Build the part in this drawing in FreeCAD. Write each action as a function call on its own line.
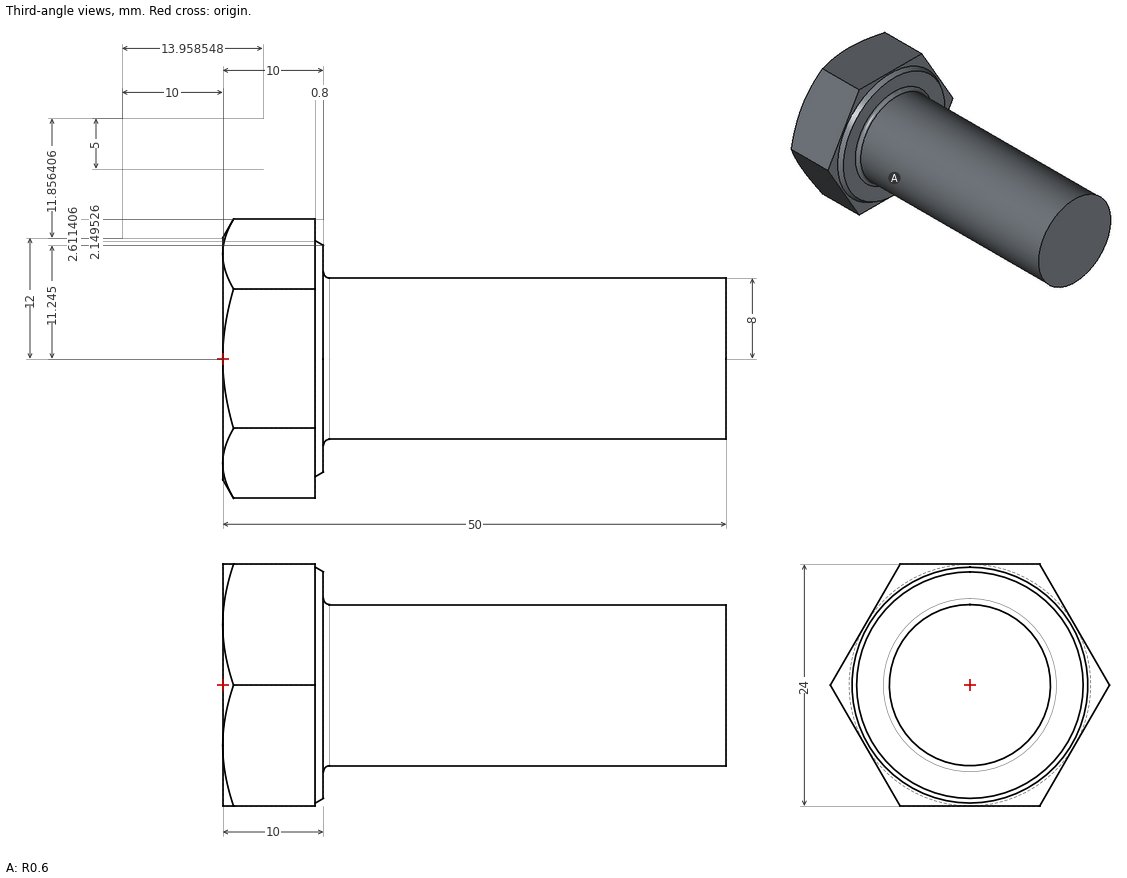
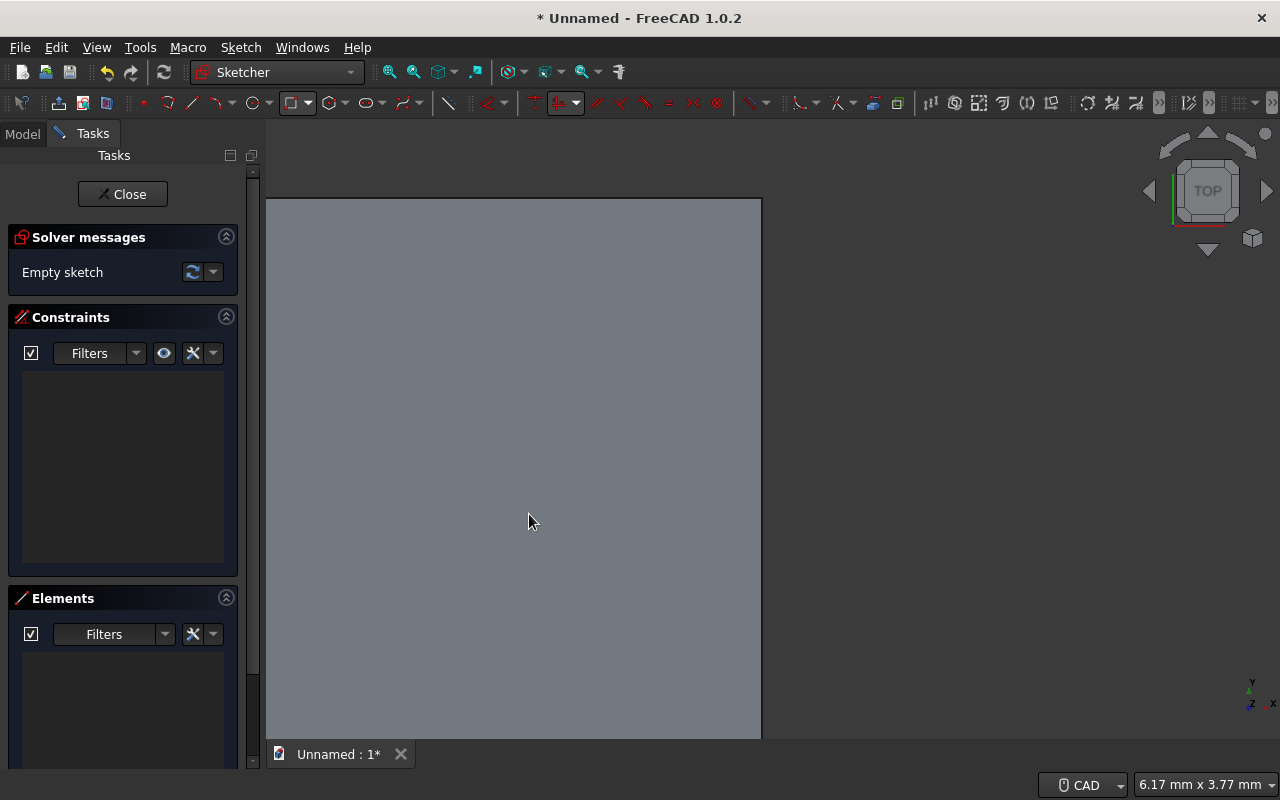
click(168, 104)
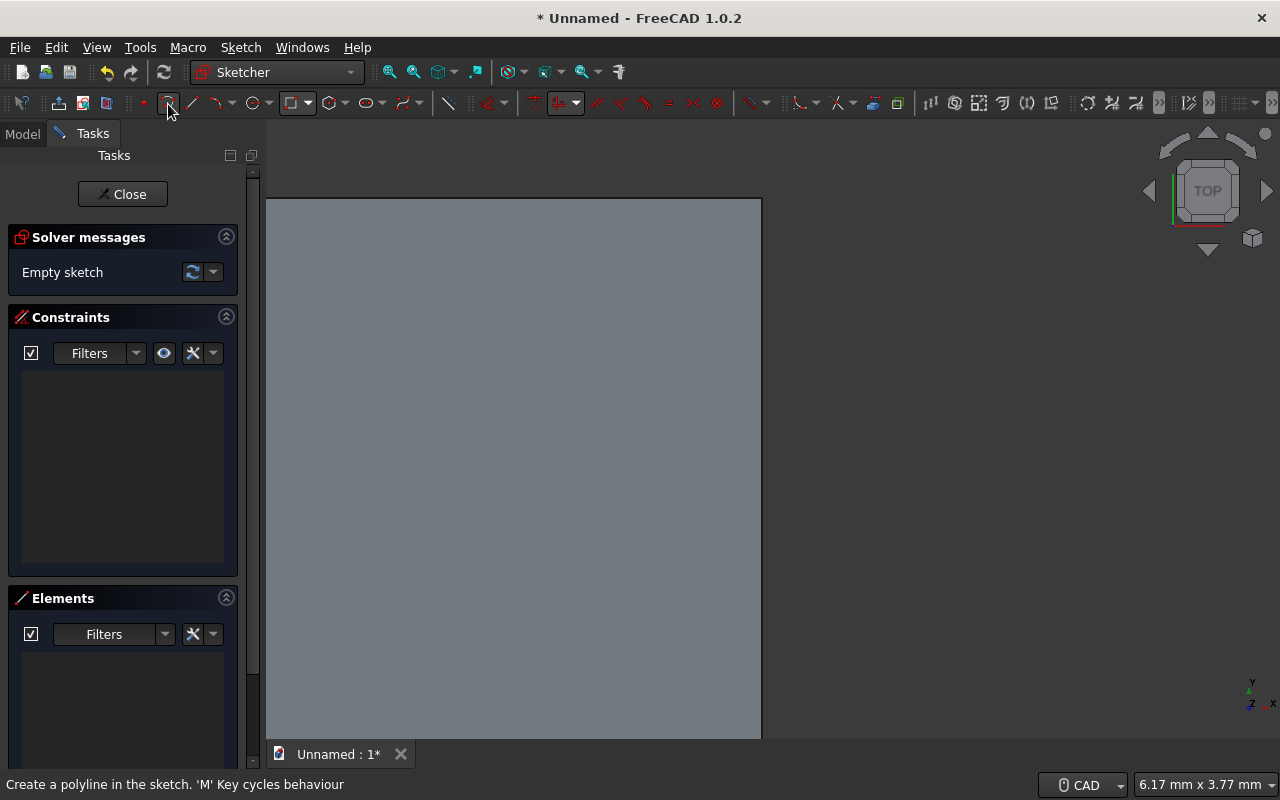
click(630, 552)
click(762, 628)
click(762, 198)
click(630, 198)
click(630, 553)
key(Escape)
key(Escape)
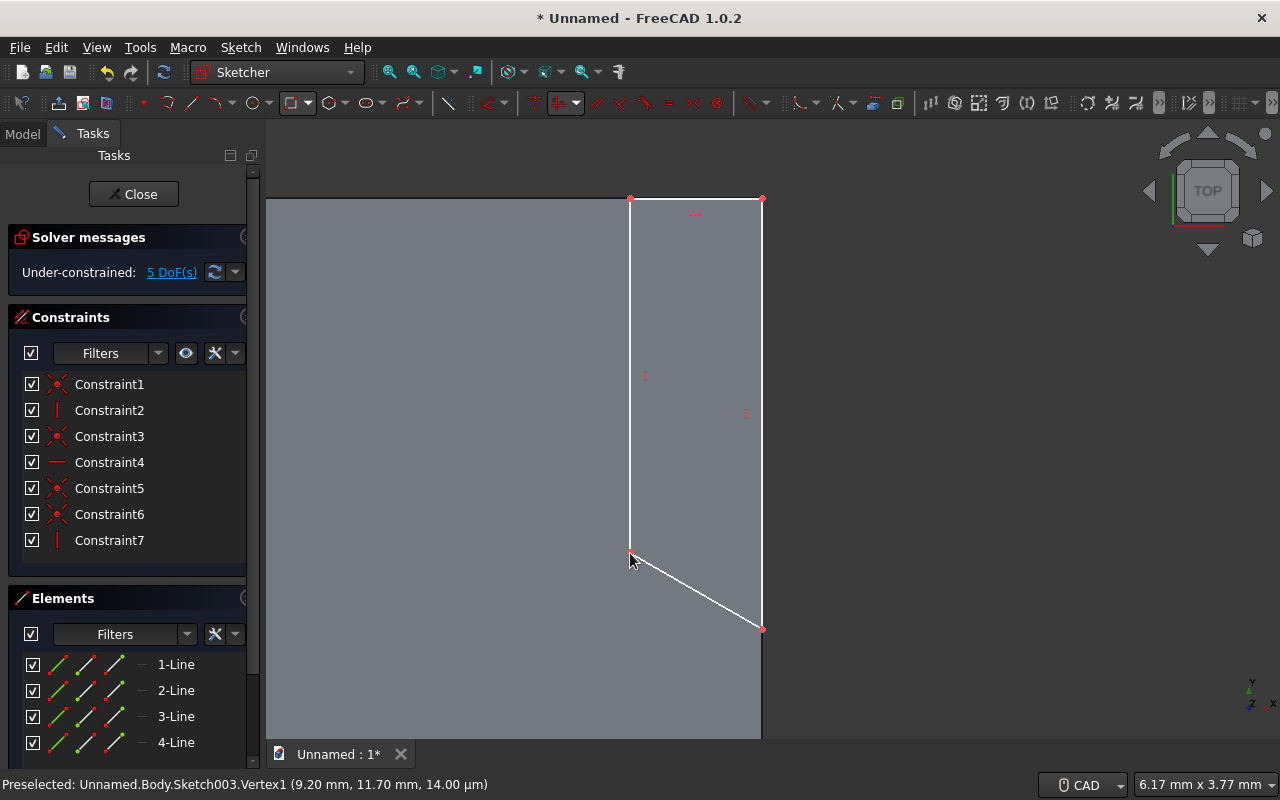
click(488, 104)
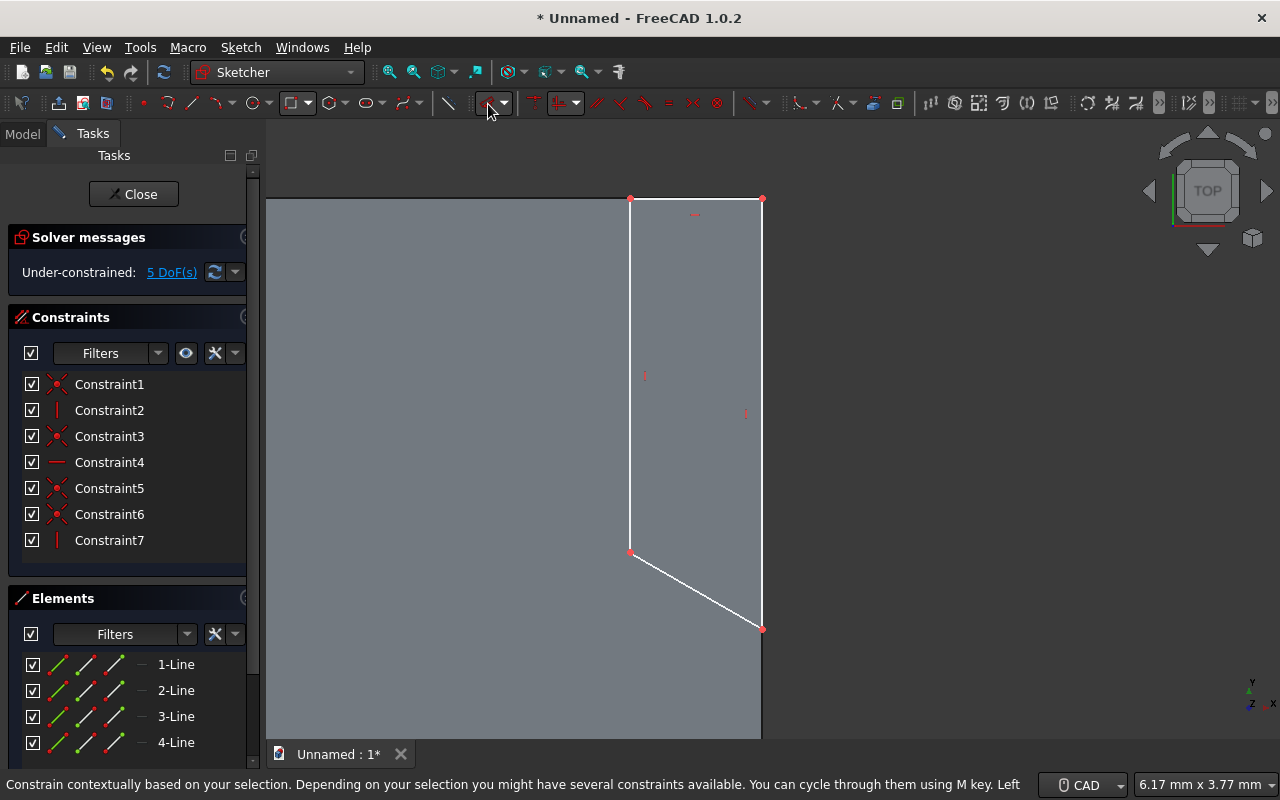
click(722, 199)
click(696, 165)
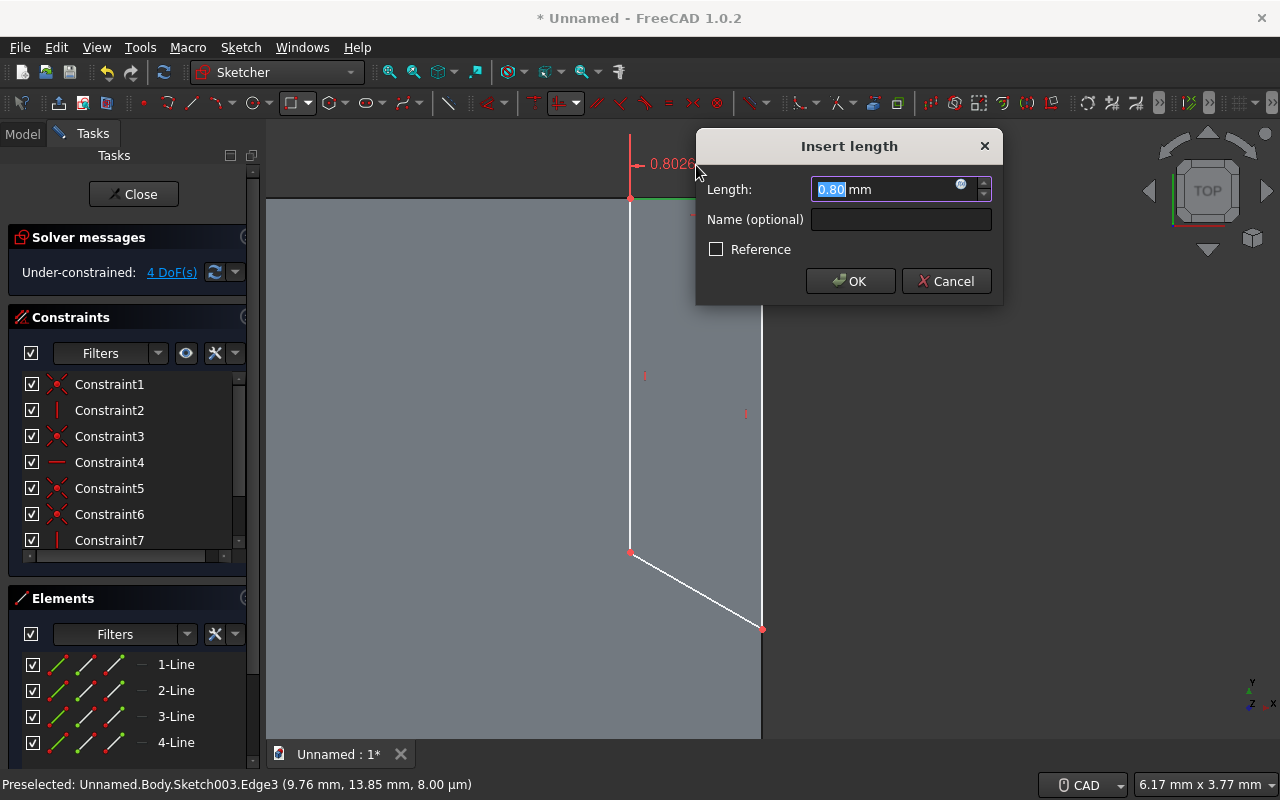
text(0.8)
key(Return)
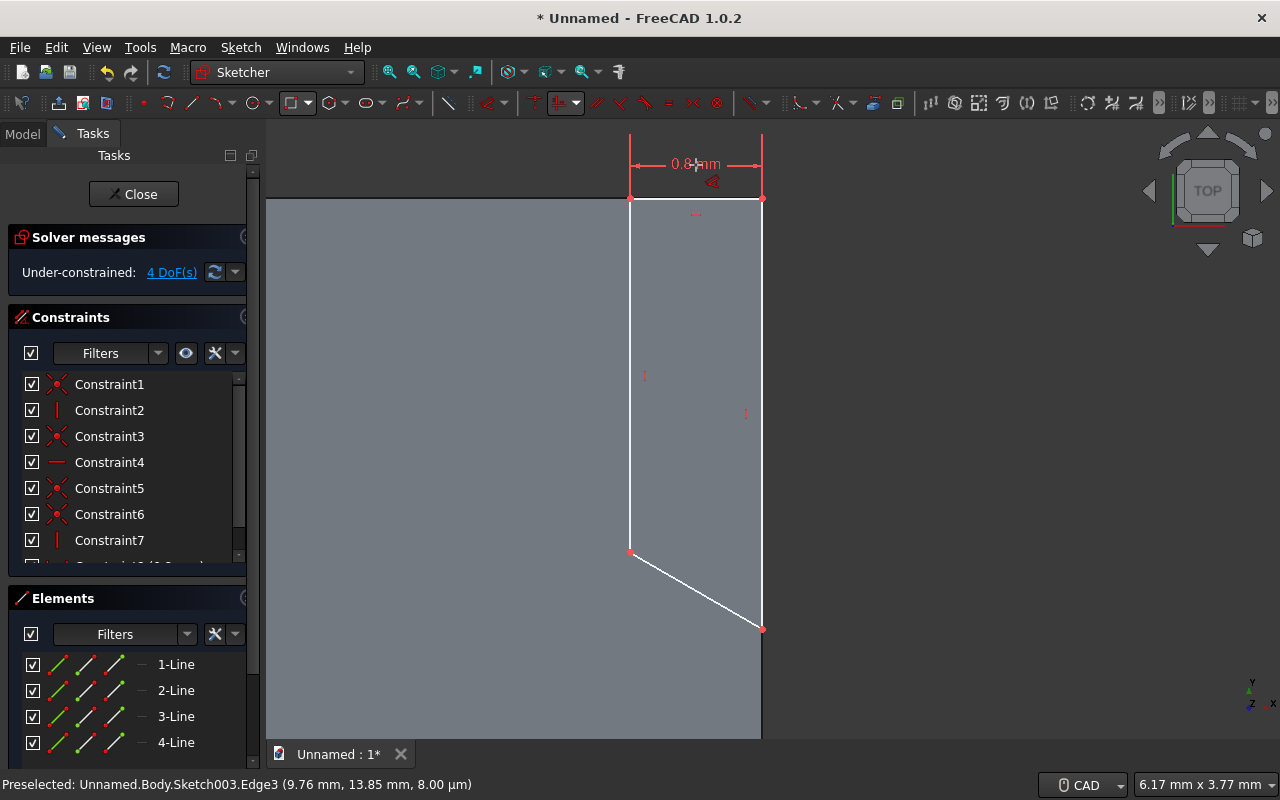
click(762, 629)
click(528, 595)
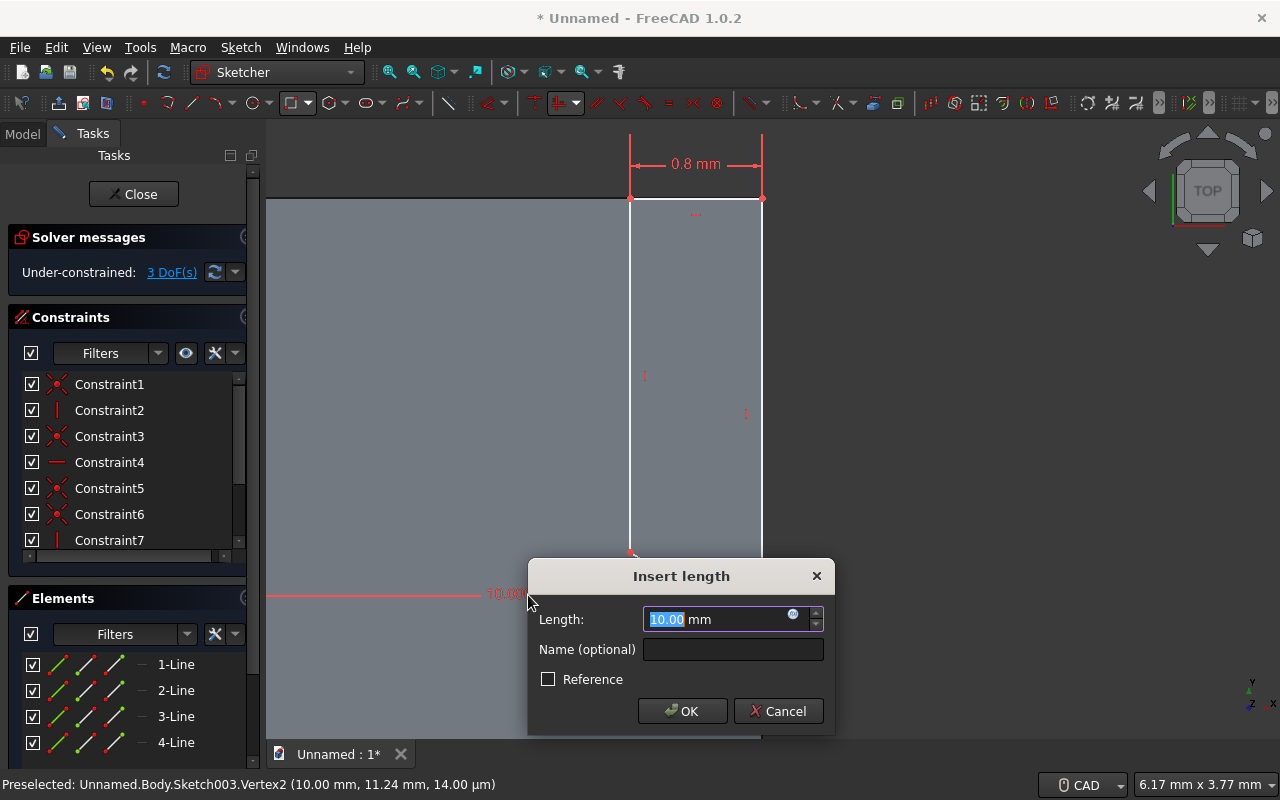
text(10)
key(Return)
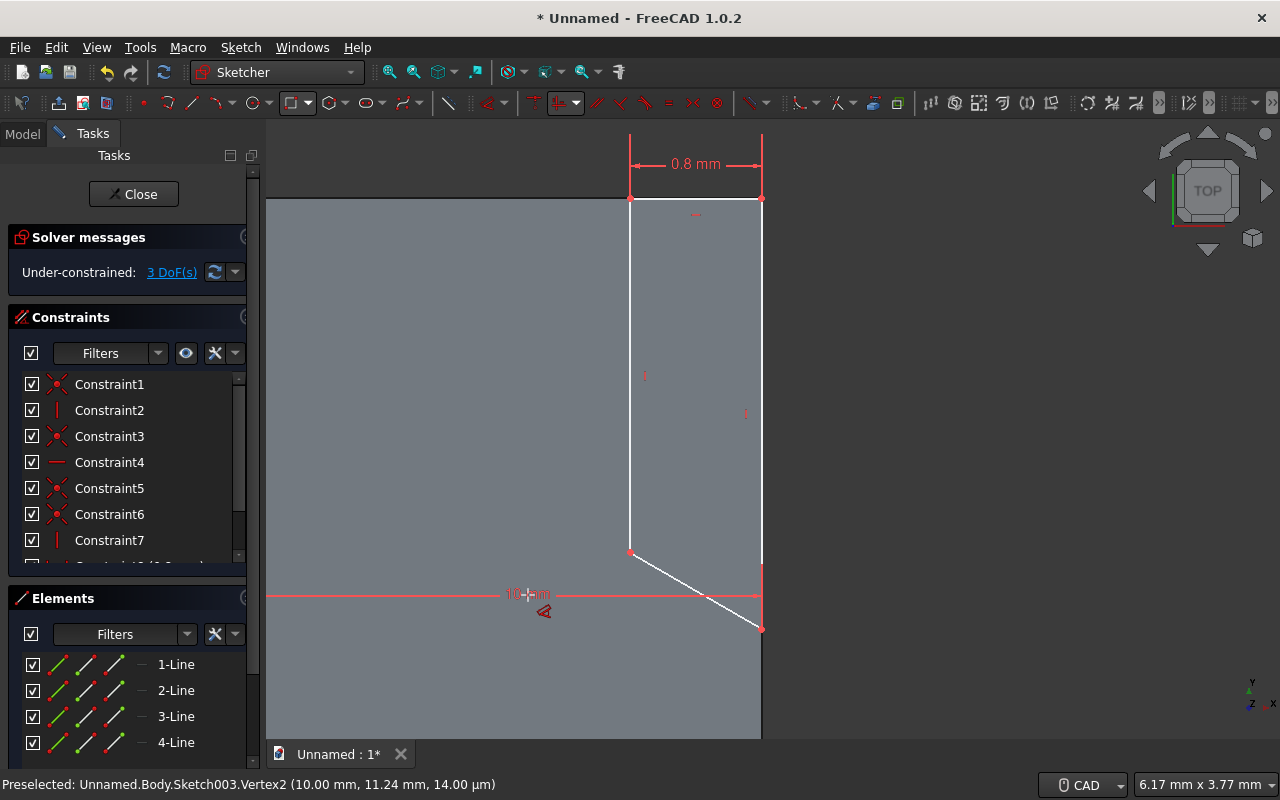
click(762, 629)
click(796, 670)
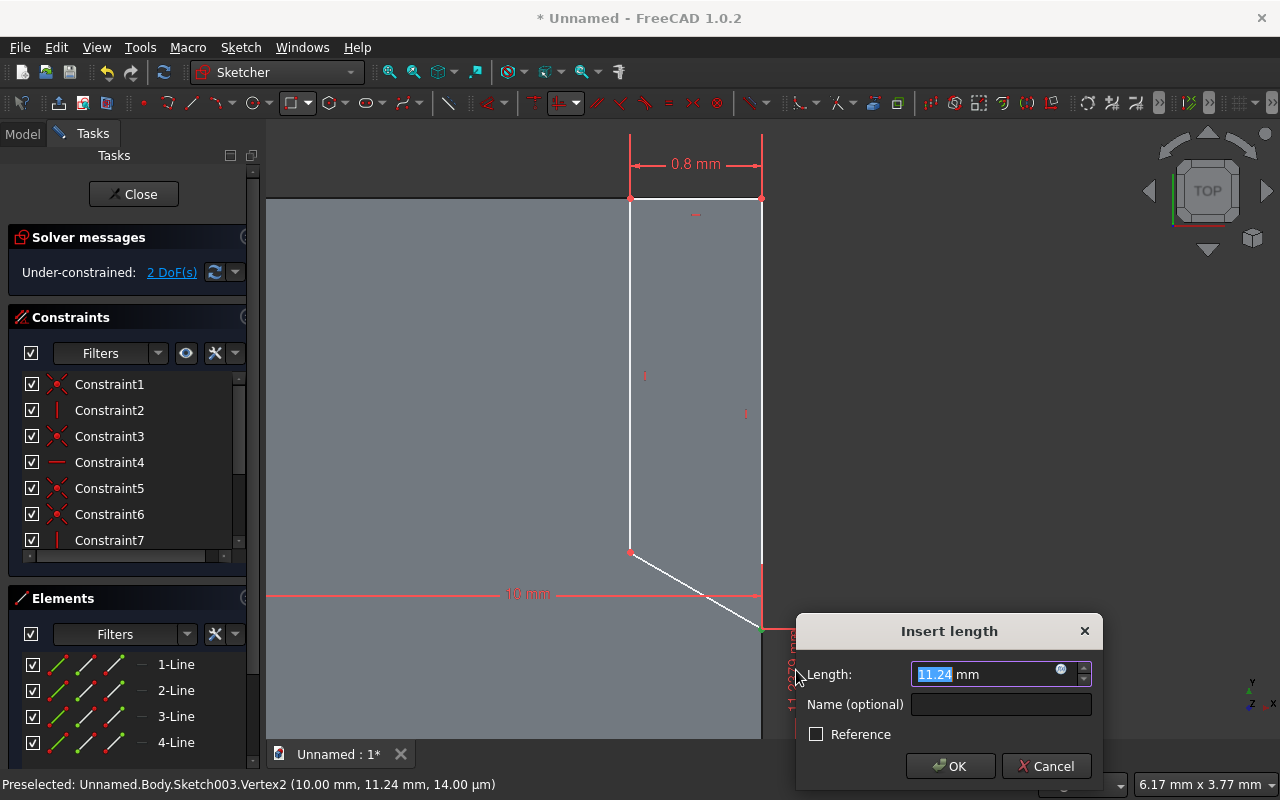
text(11.245)
key(Return)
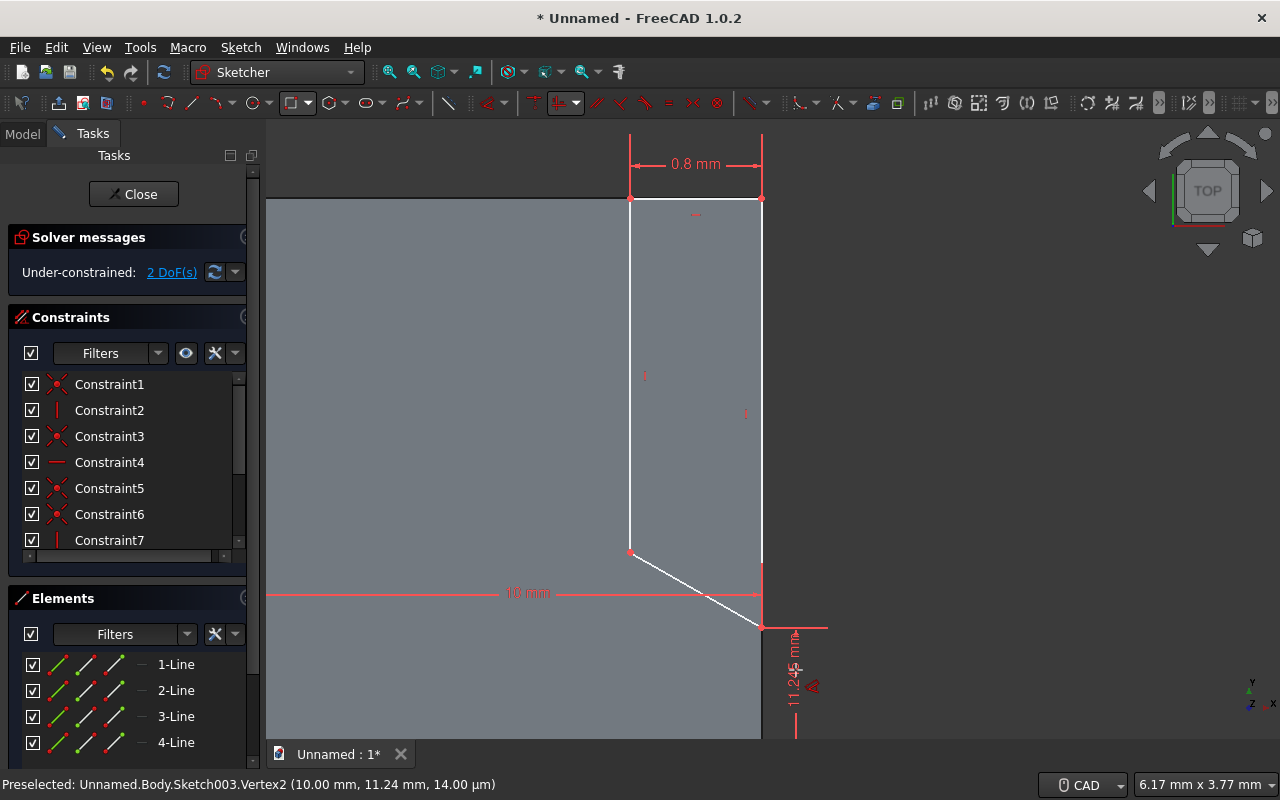
click(762, 499)
click(796, 413)